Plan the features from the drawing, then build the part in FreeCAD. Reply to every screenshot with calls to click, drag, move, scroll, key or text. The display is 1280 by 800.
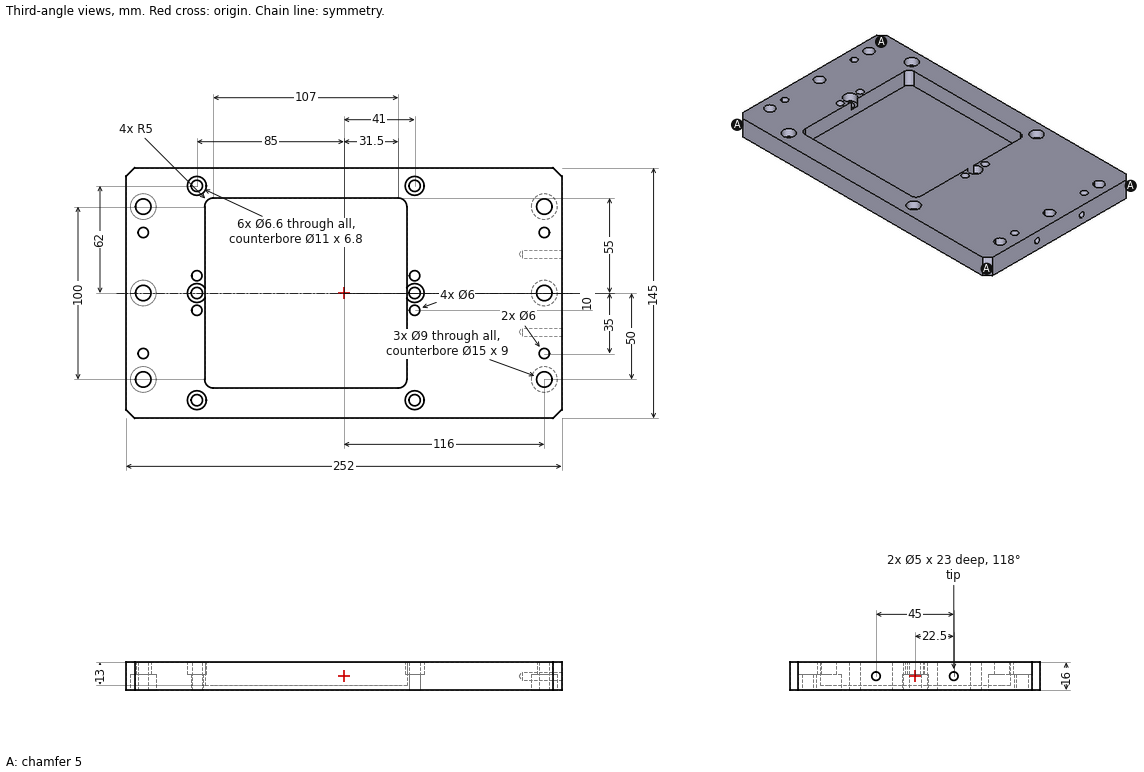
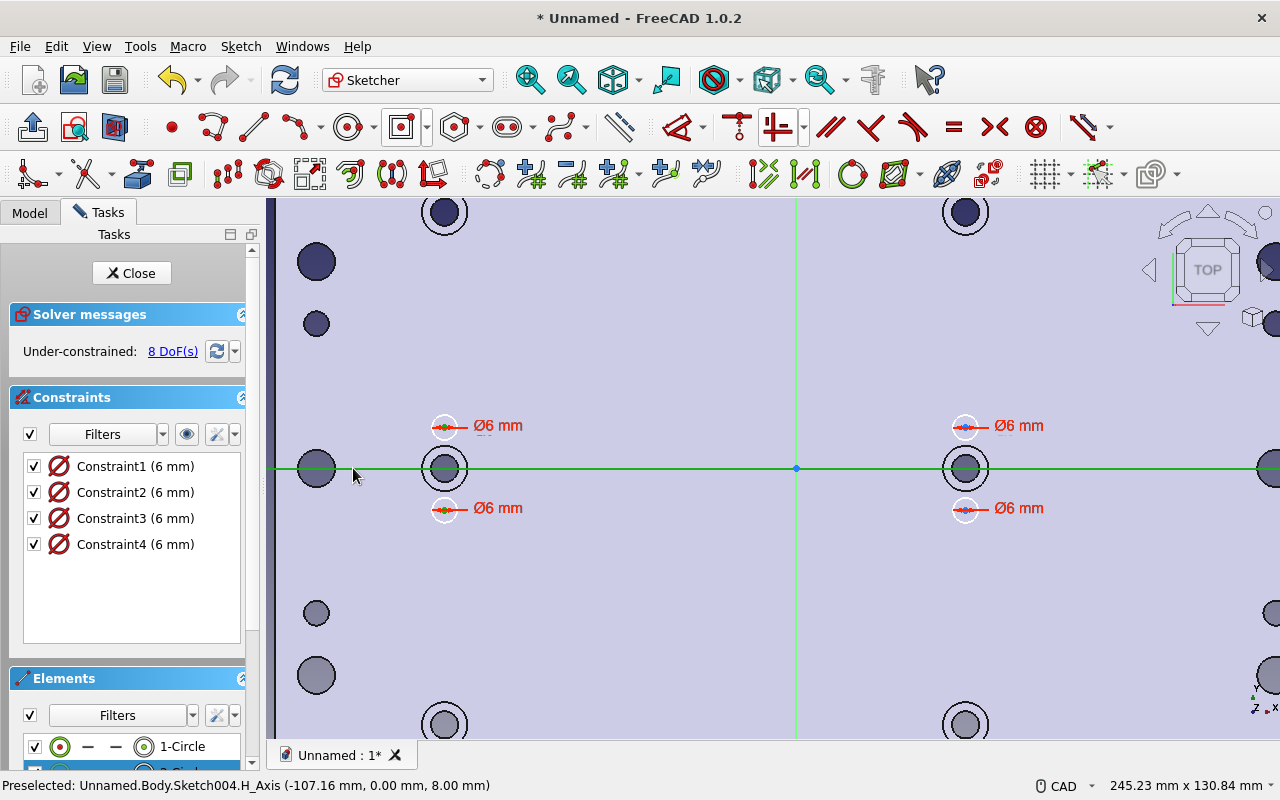
key(s)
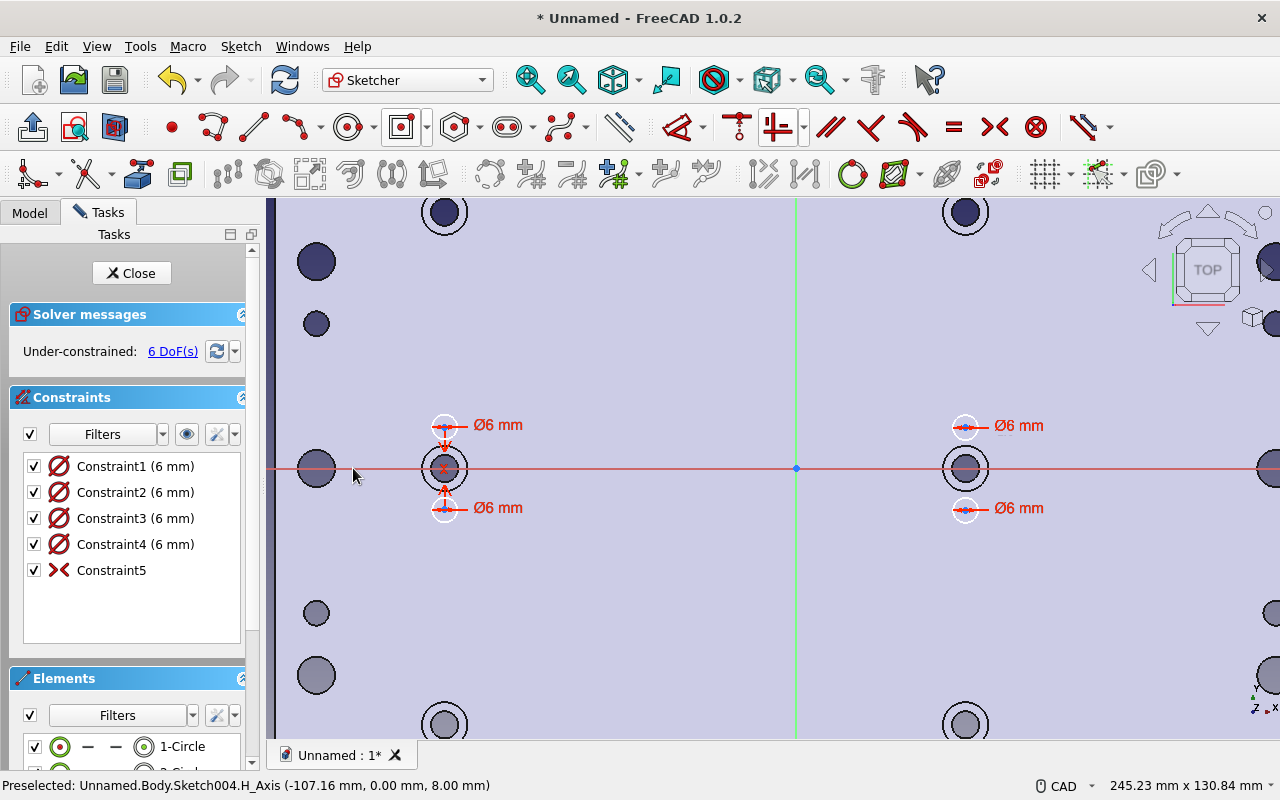
click(966, 510)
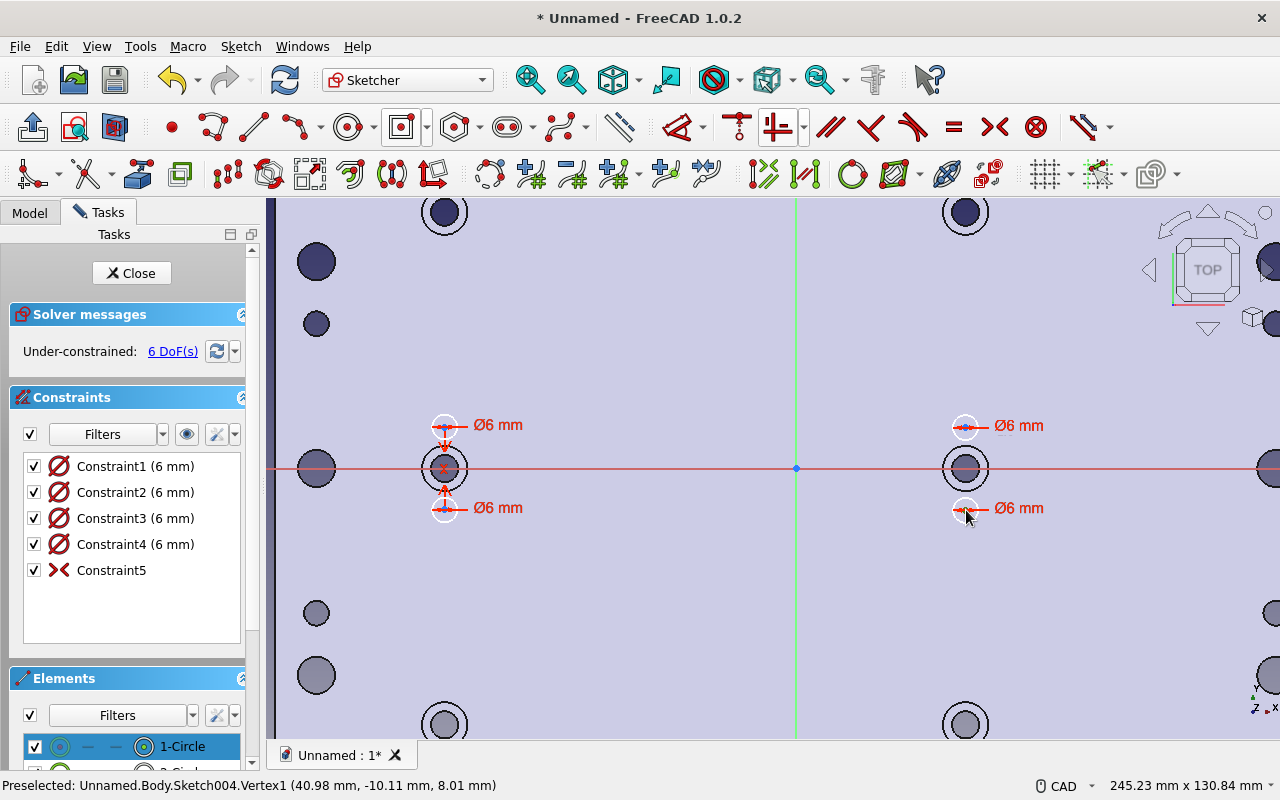
click(965, 428)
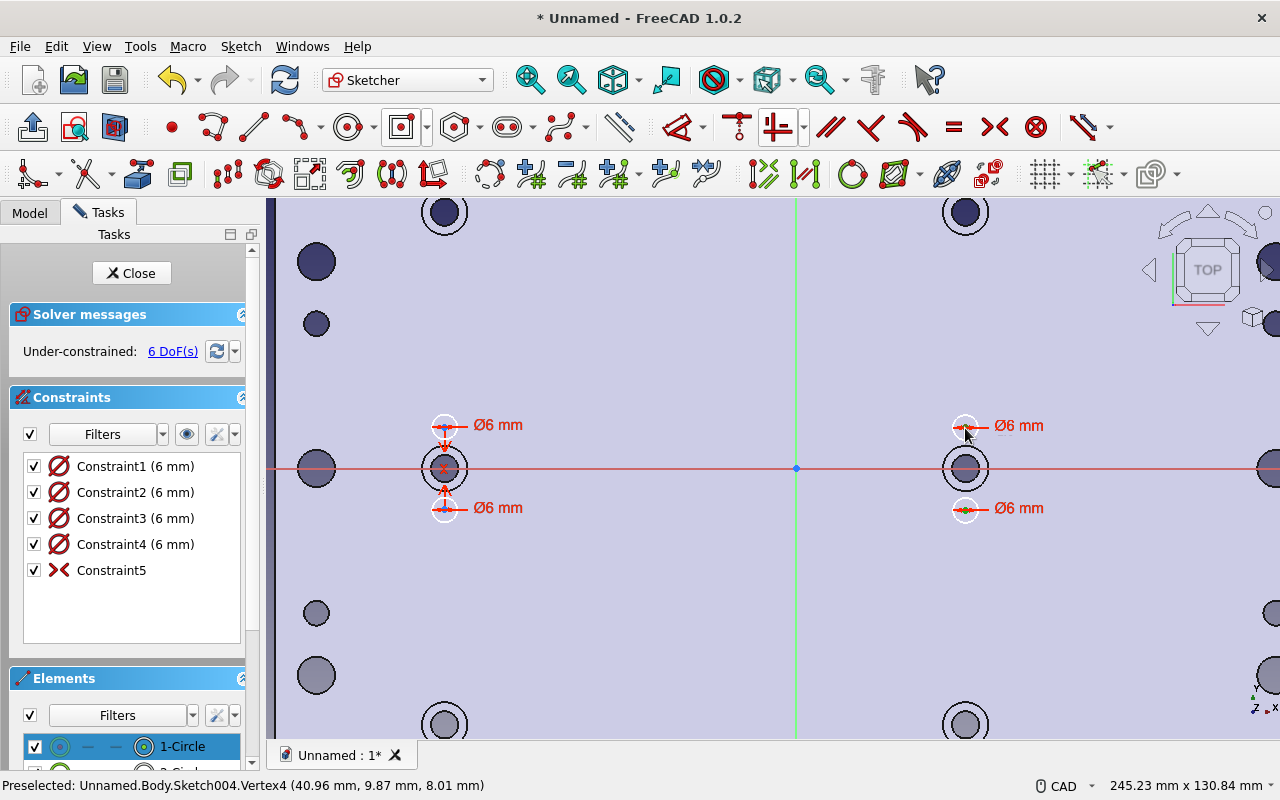
click(353, 468)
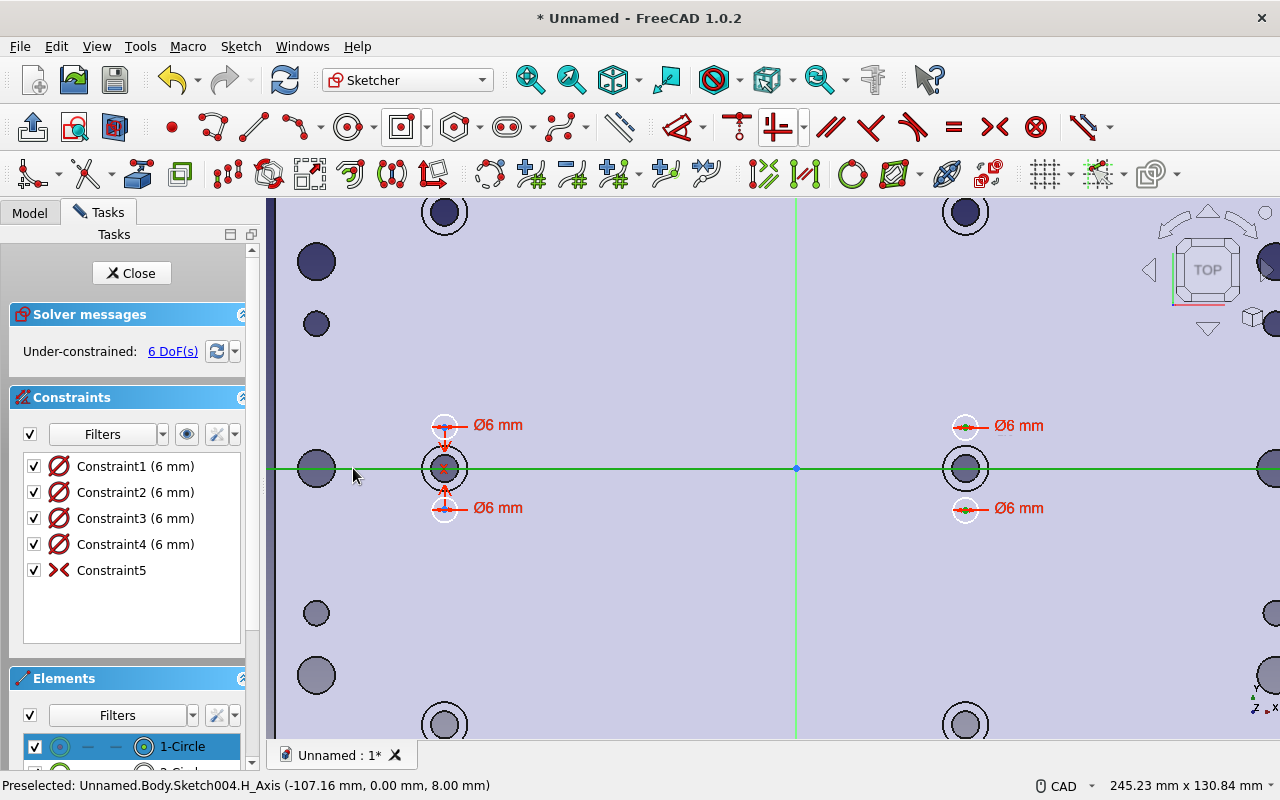
key(s)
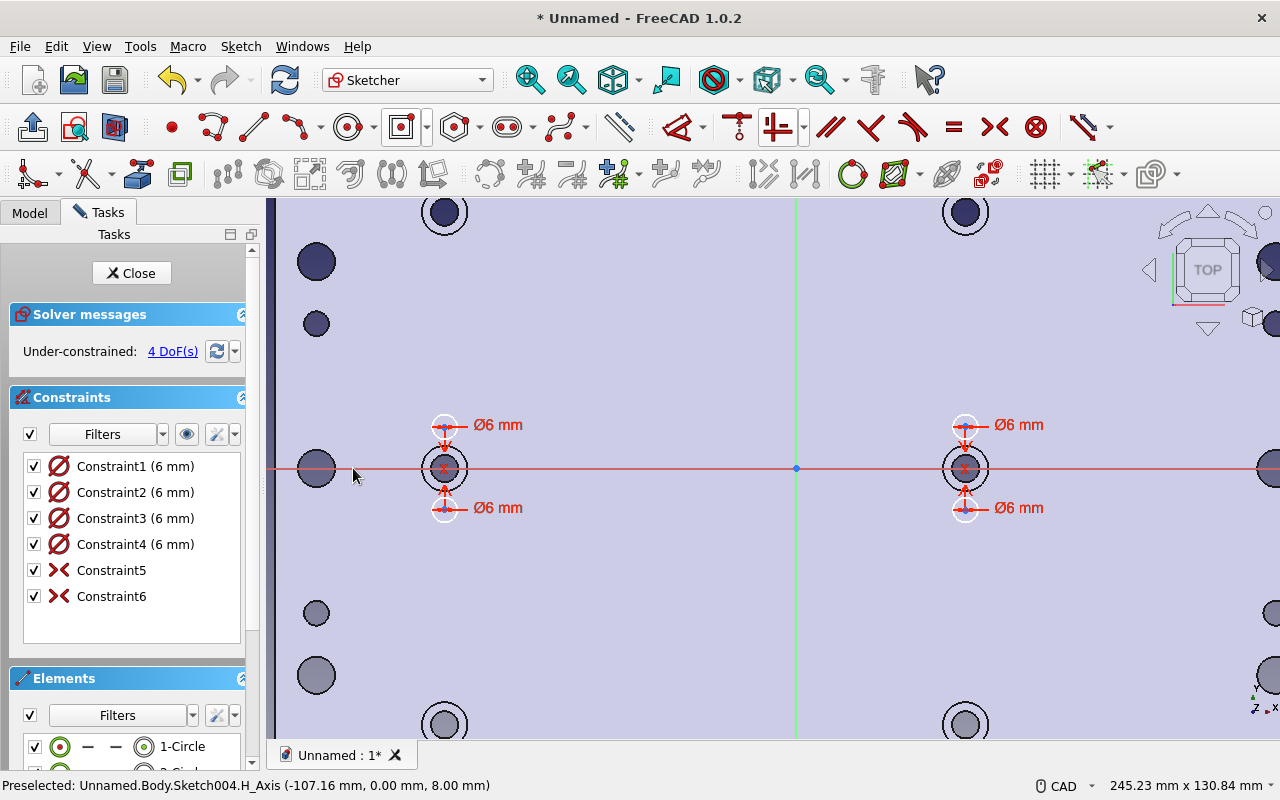
click(676, 128)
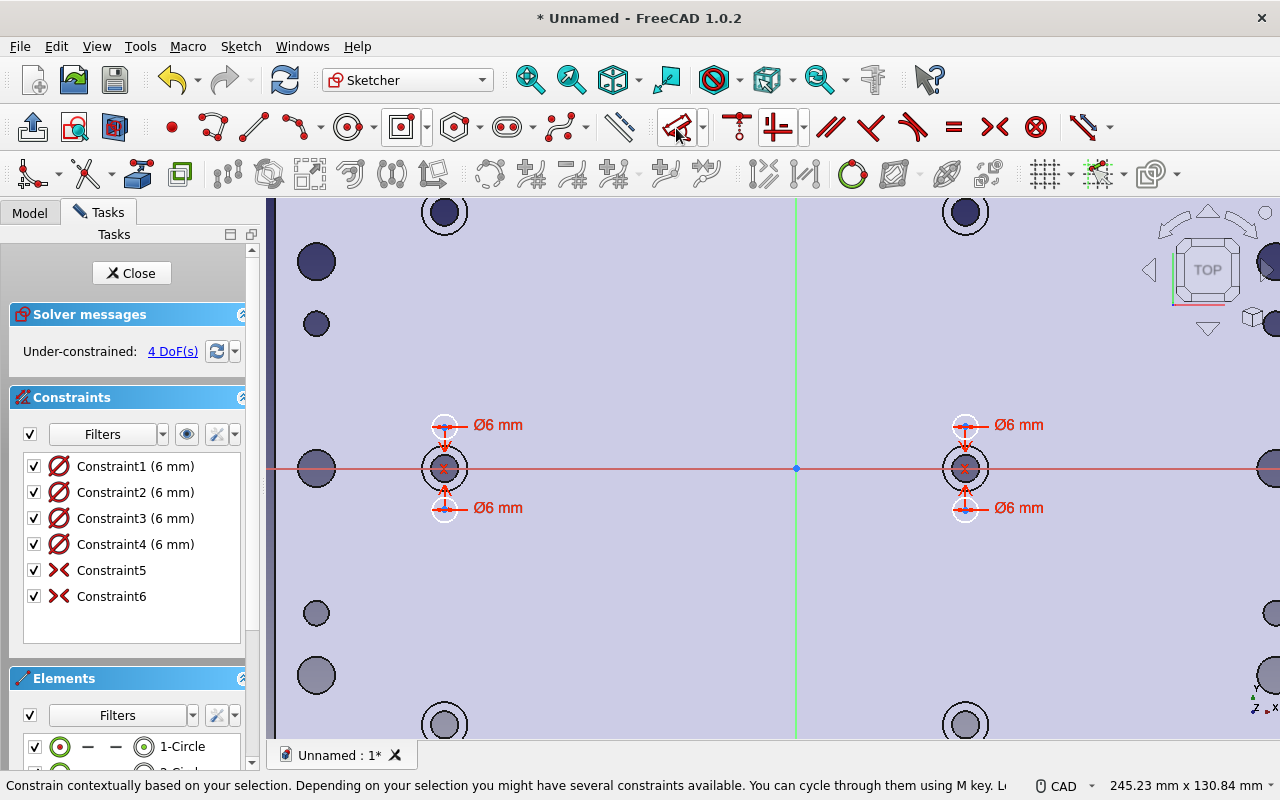
click(965, 510)
click(881, 544)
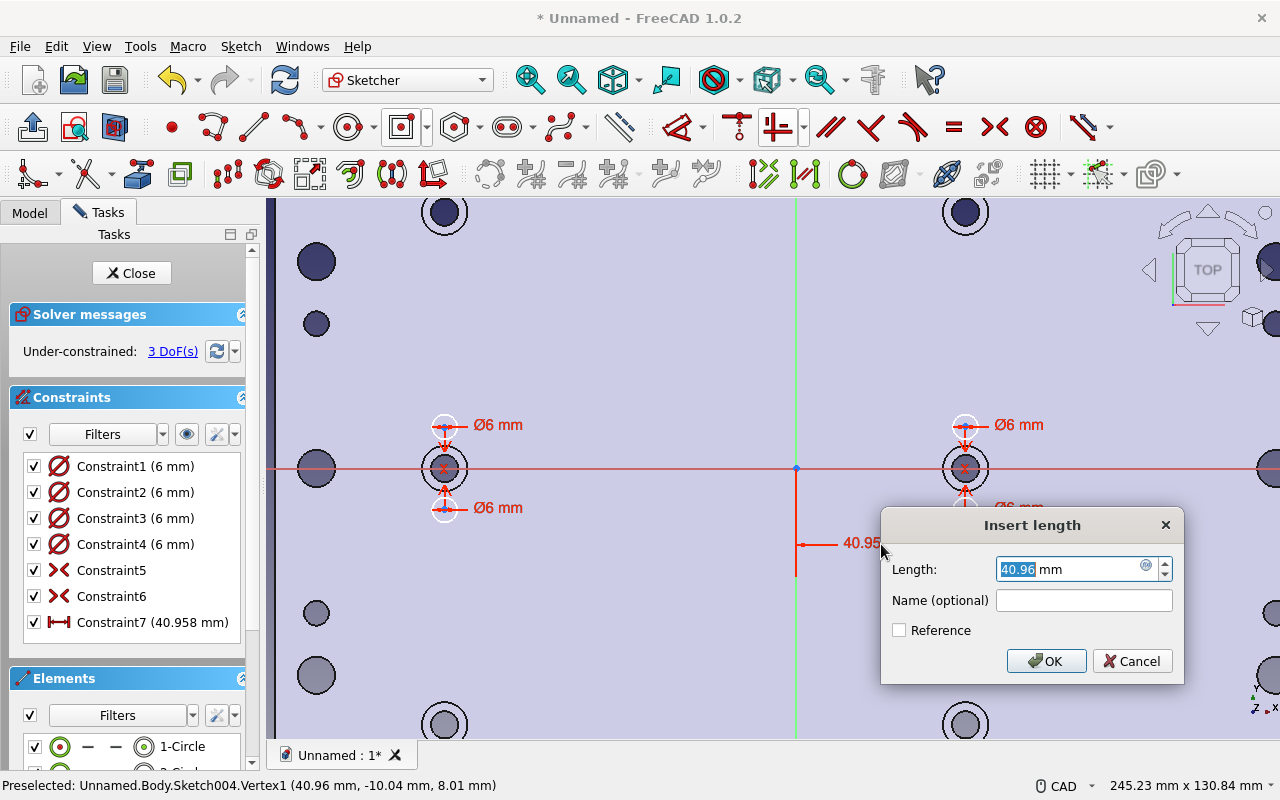
text(41)
key(Return)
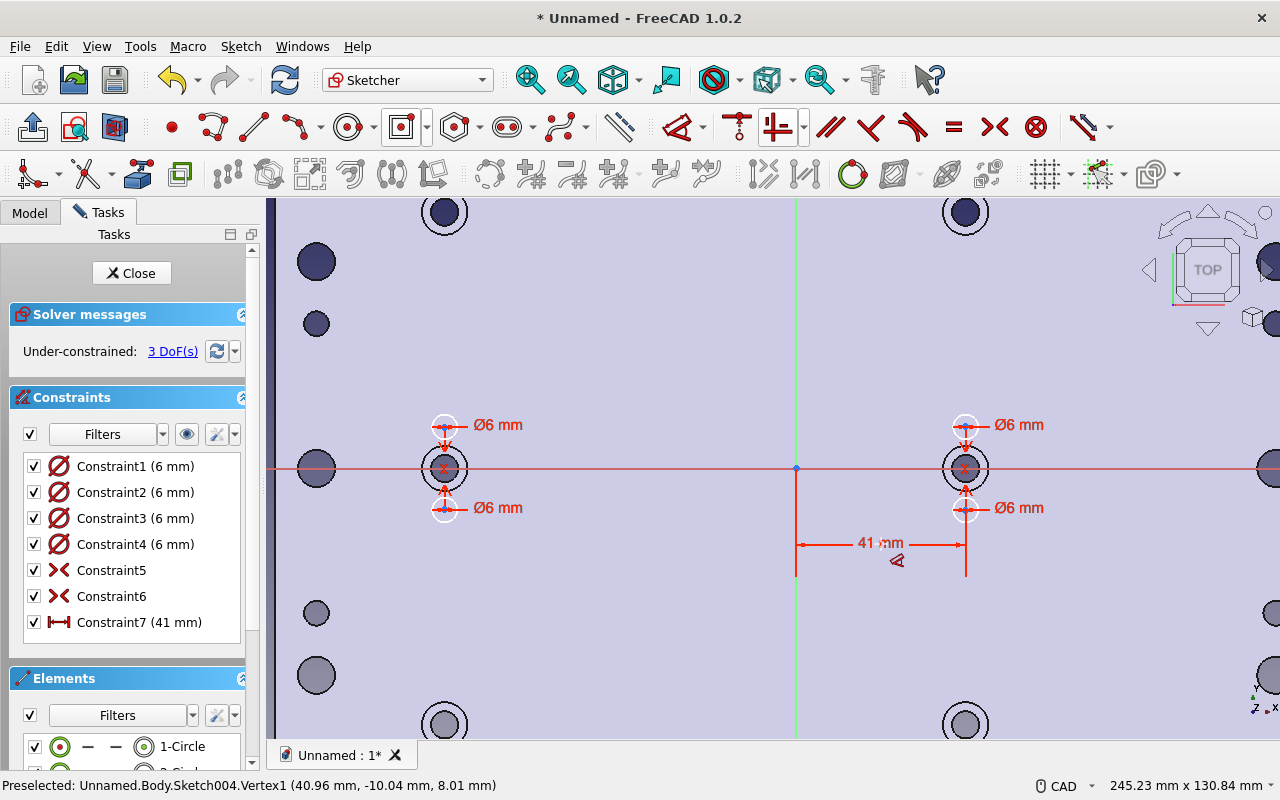
click(966, 510)
click(1000, 489)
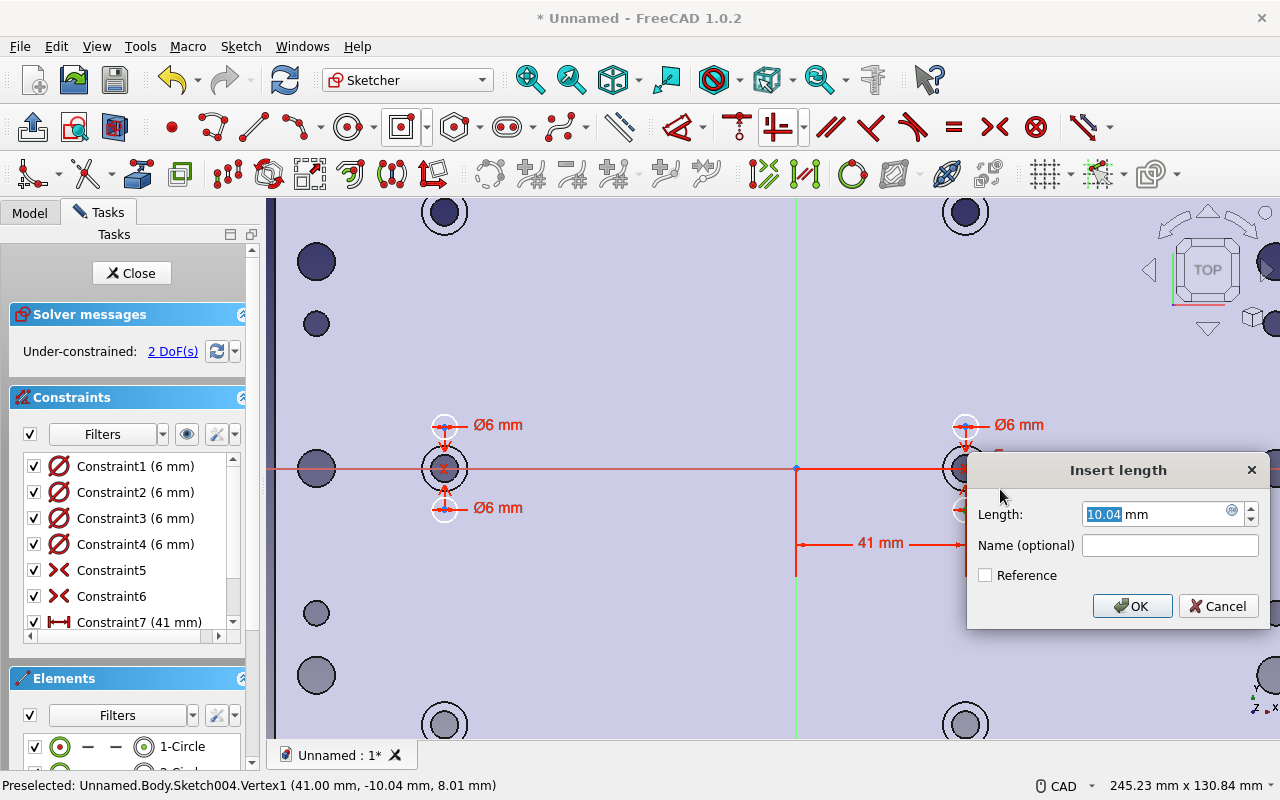
text(10)
key(Return)